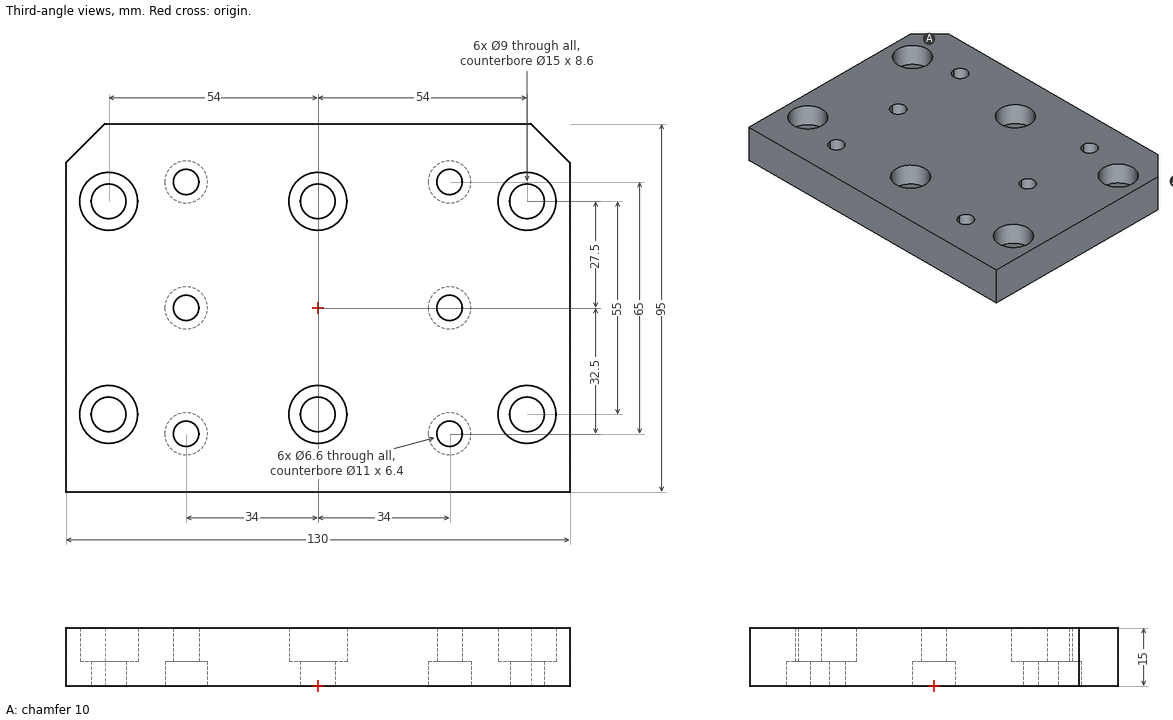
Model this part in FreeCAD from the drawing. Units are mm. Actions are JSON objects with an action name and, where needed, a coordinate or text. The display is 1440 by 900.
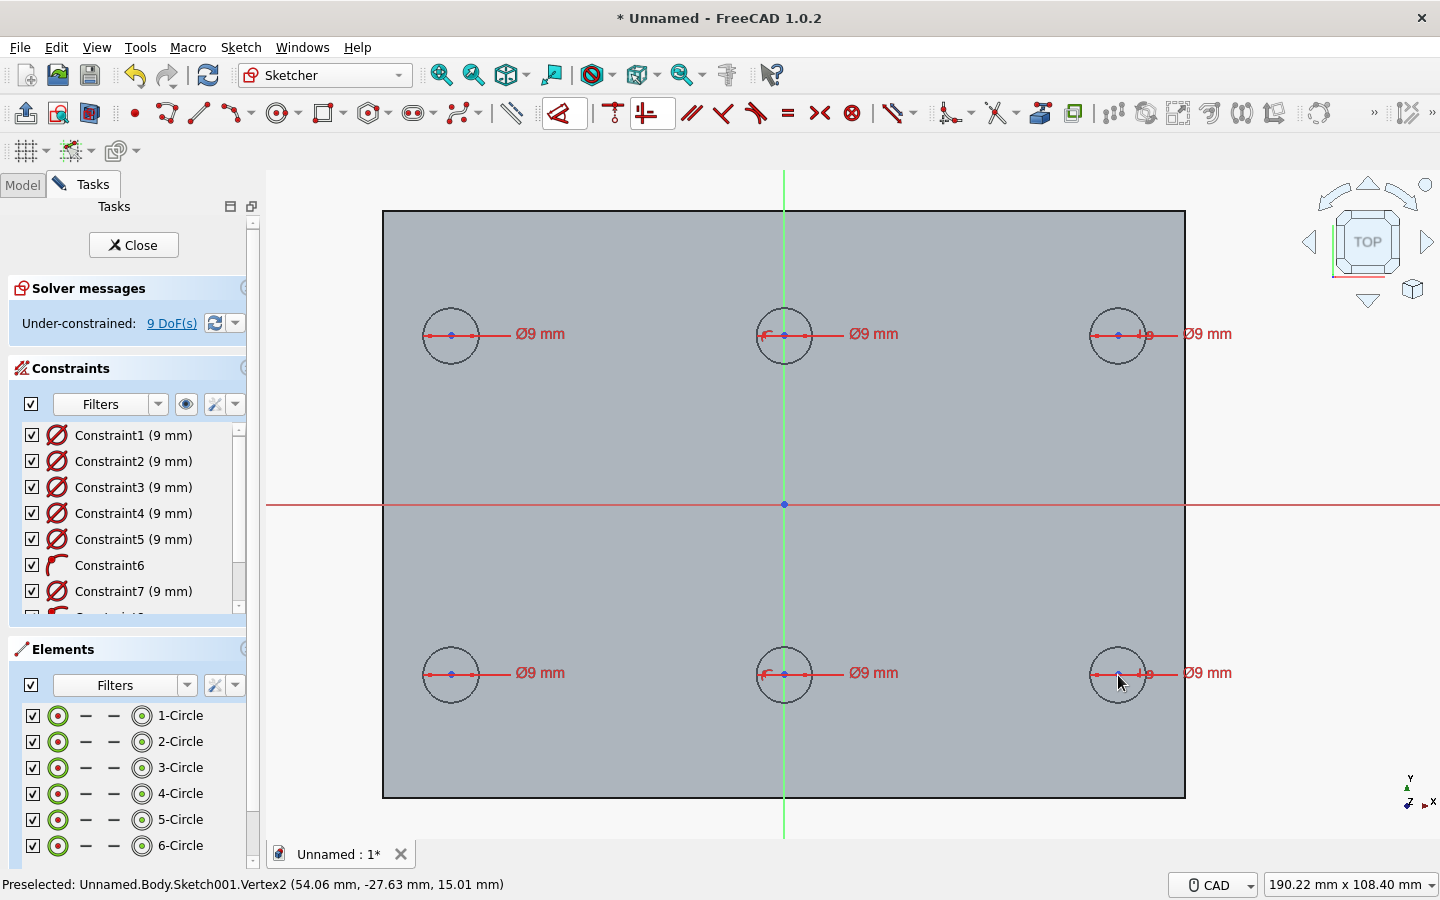
{"action": "left_click", "coordinate": [1118, 336]}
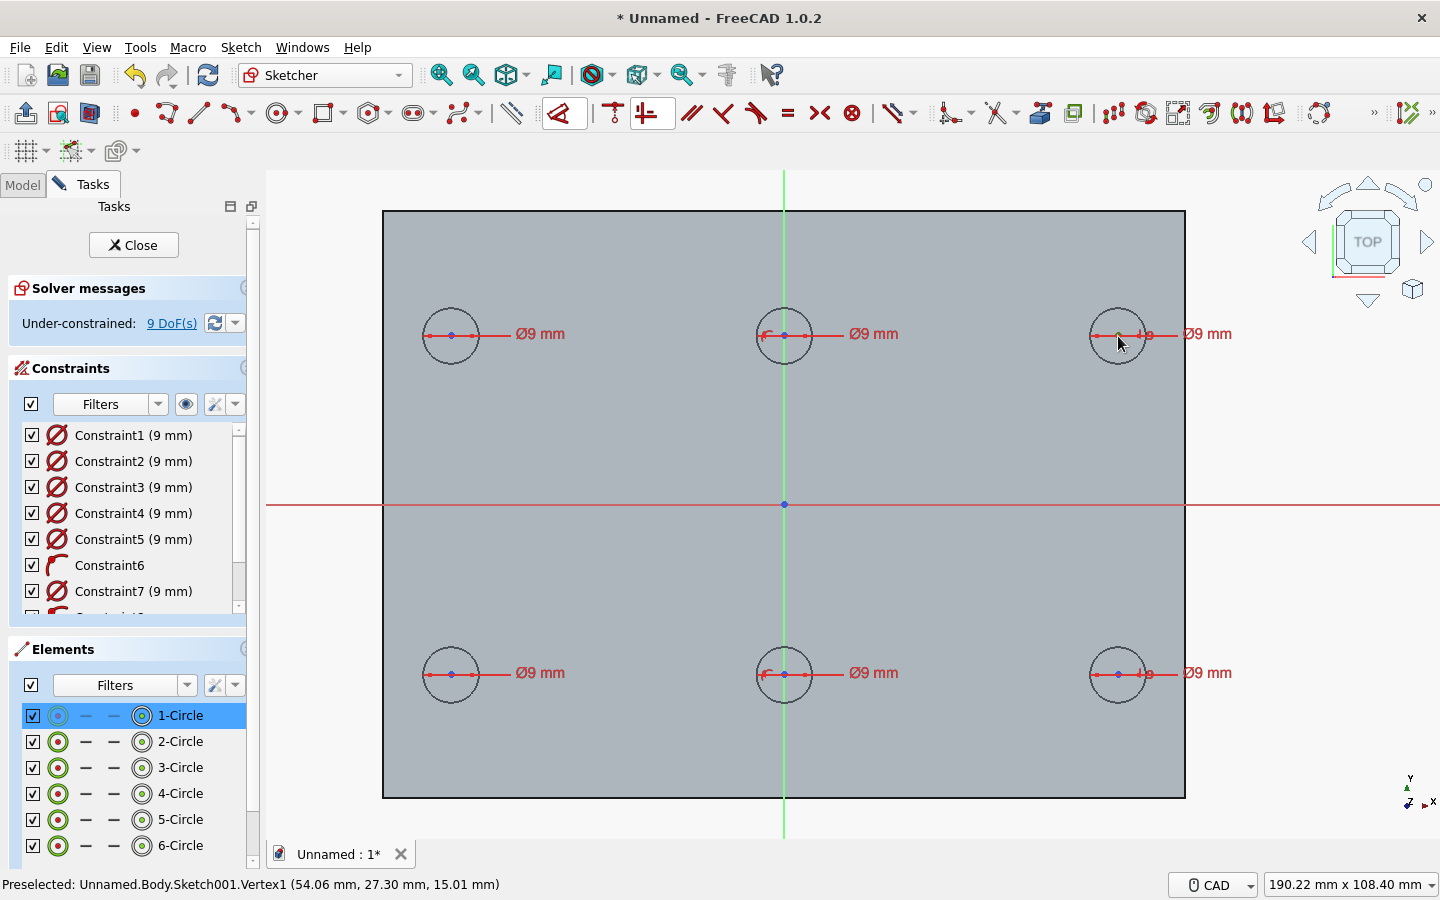
{"action": "left_click", "coordinate": [451, 336]}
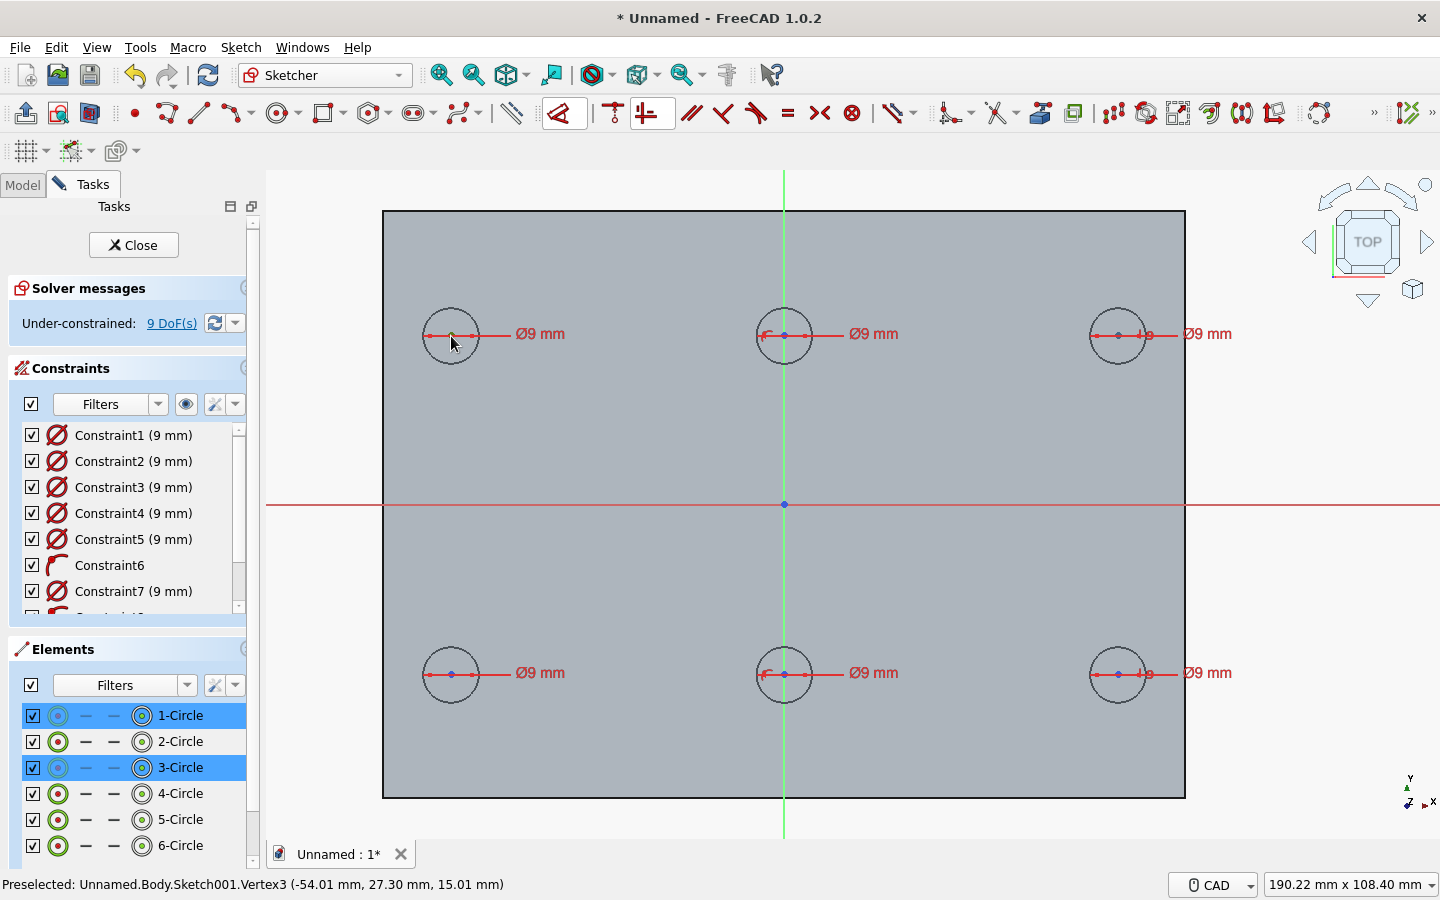
{"action": "key", "text": "h"}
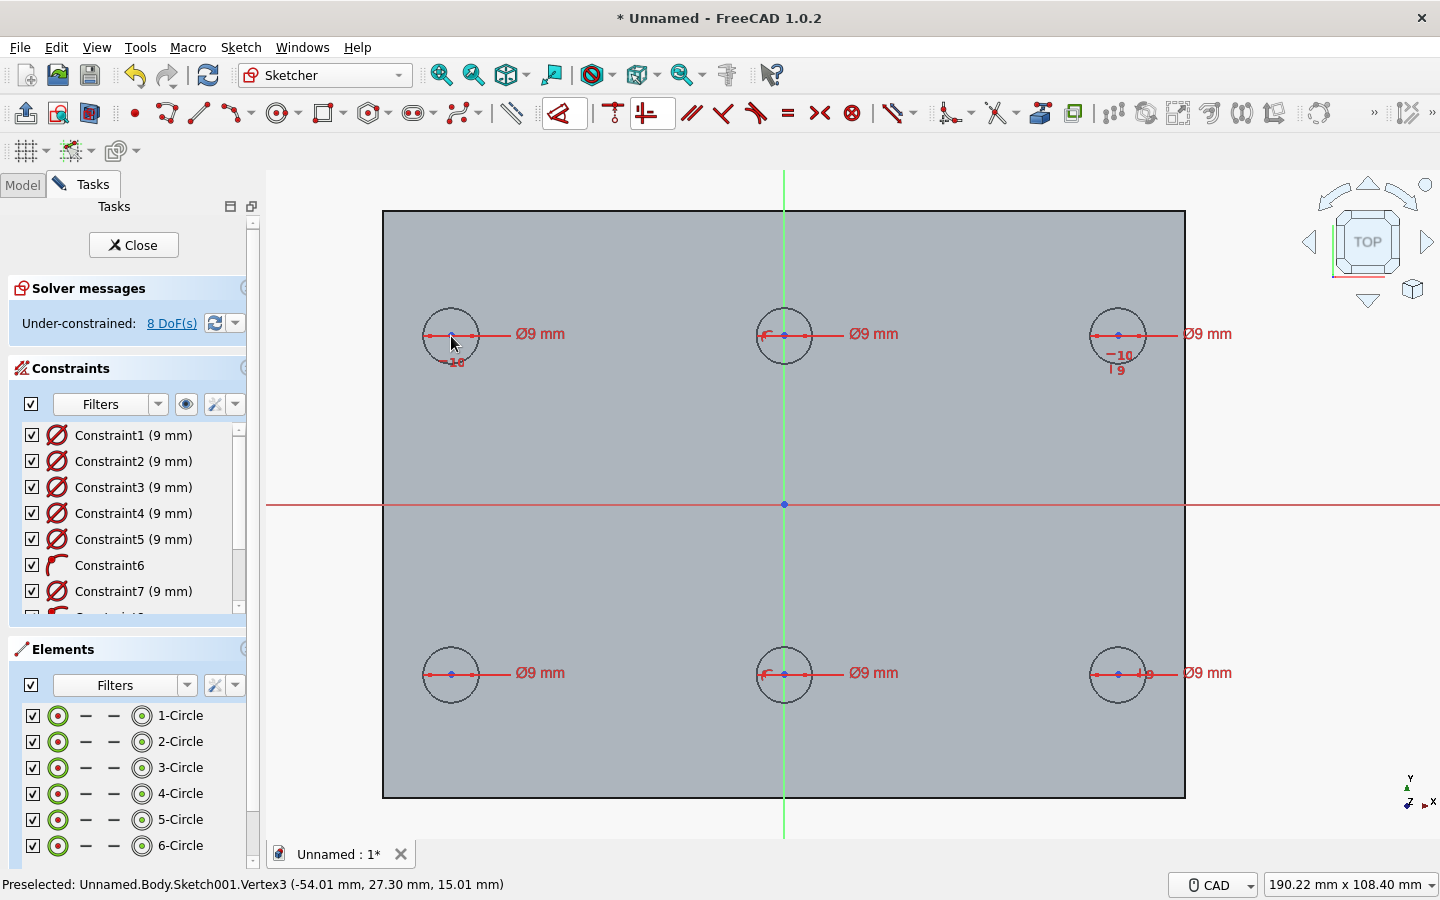
{"action": "left_click", "coordinate": [451, 336]}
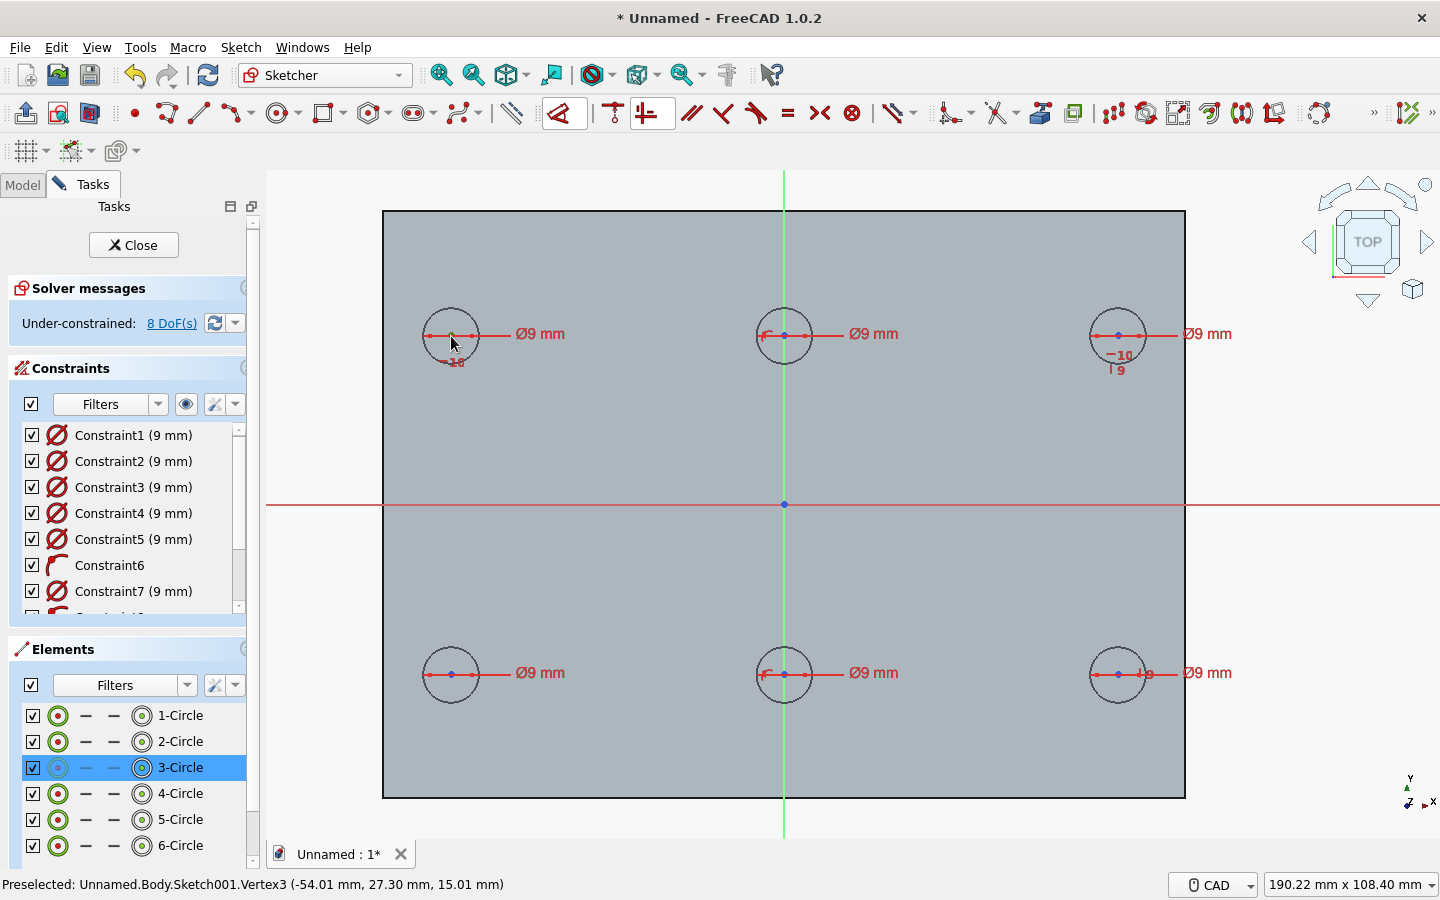
{"action": "left_click", "coordinate": [451, 675]}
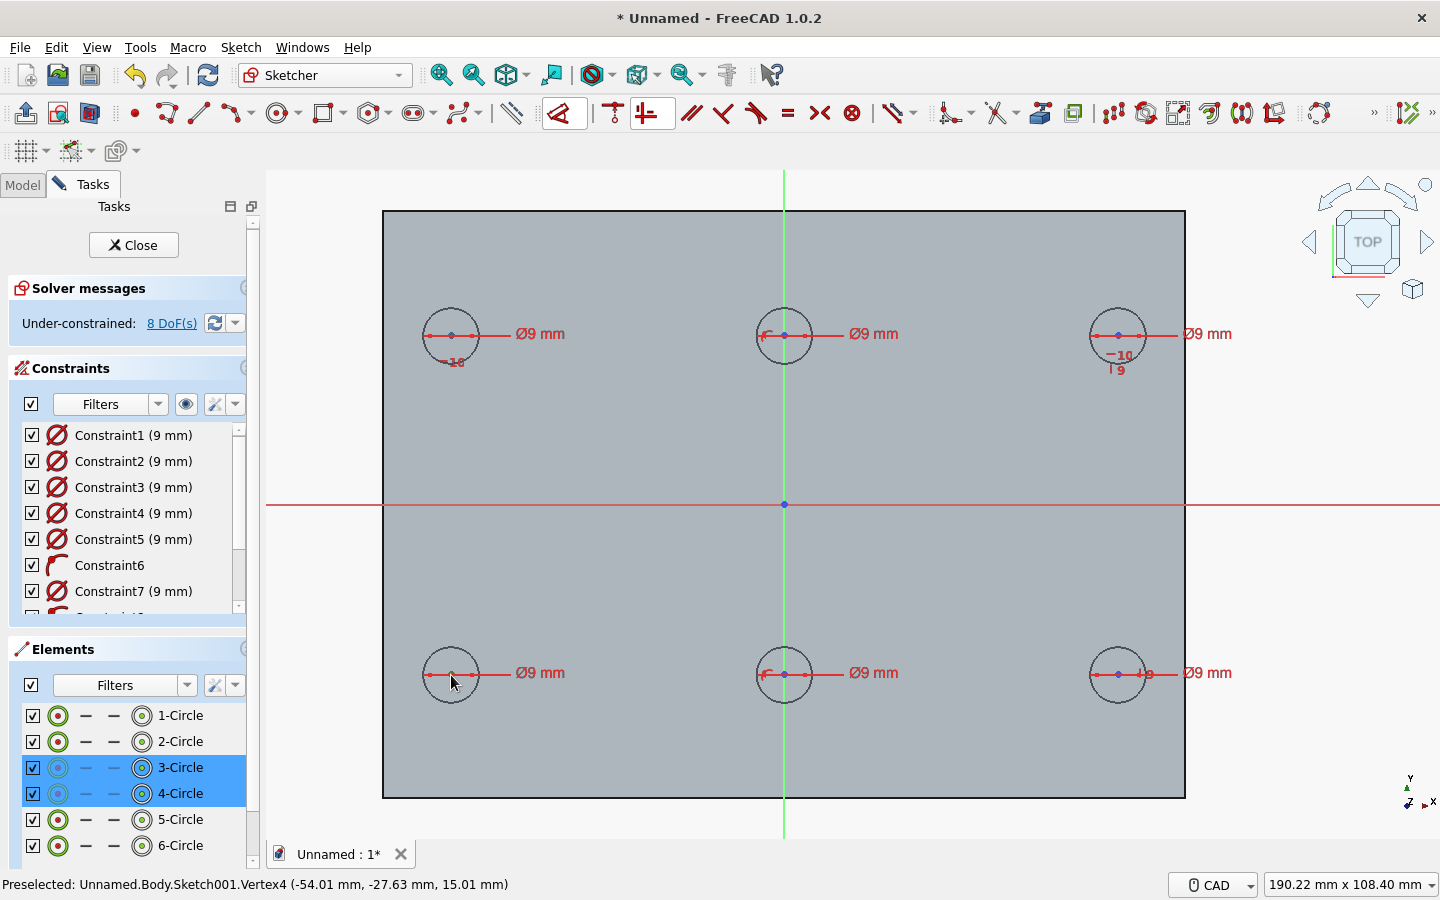
{"action": "key", "text": "v"}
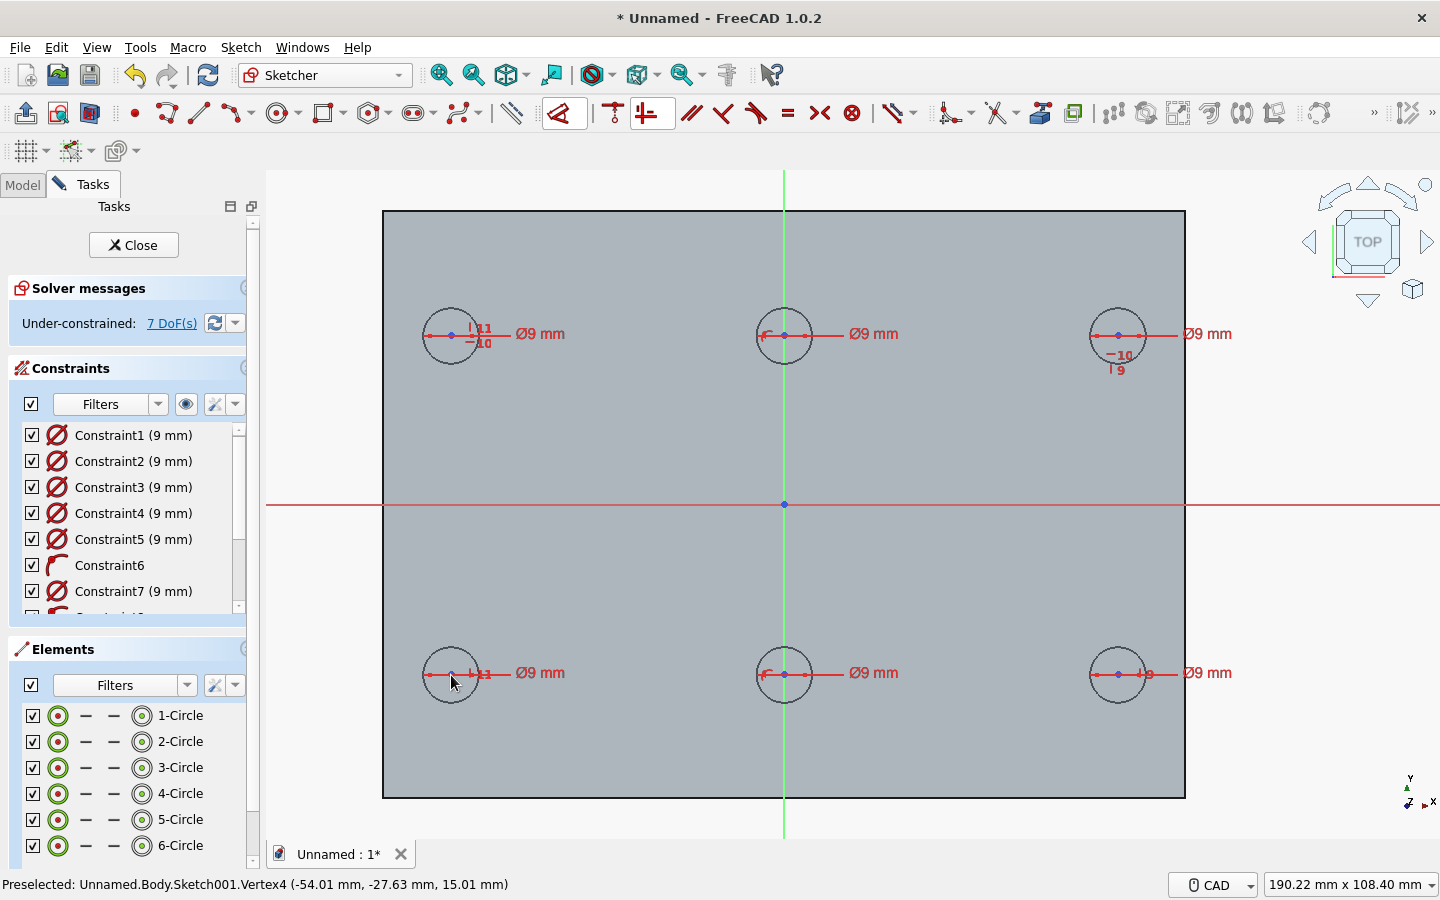
{"action": "left_click", "coordinate": [1118, 675]}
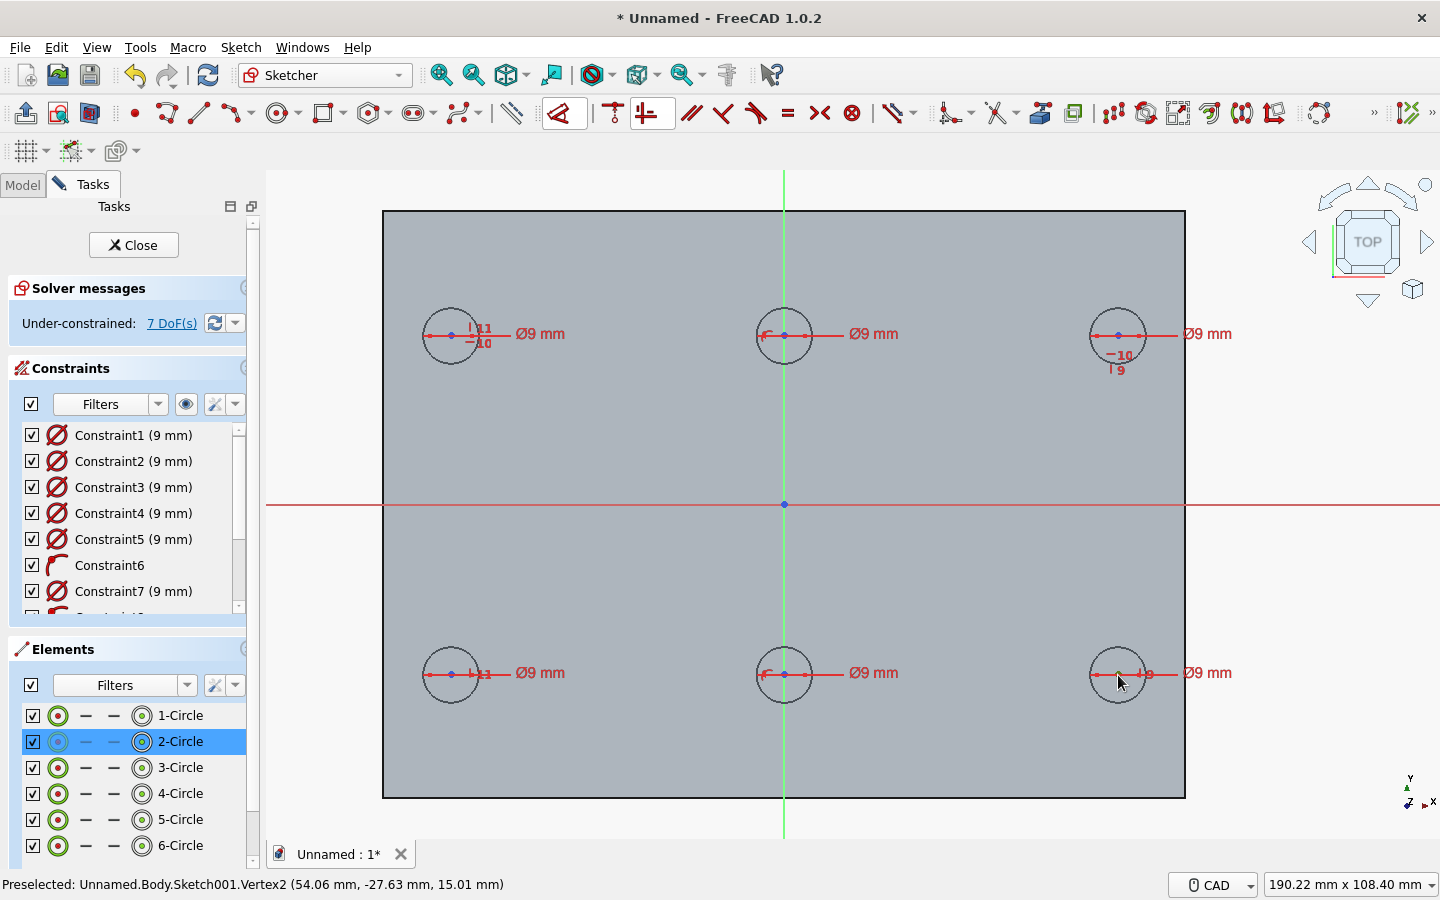
{"action": "left_click", "coordinate": [451, 675]}